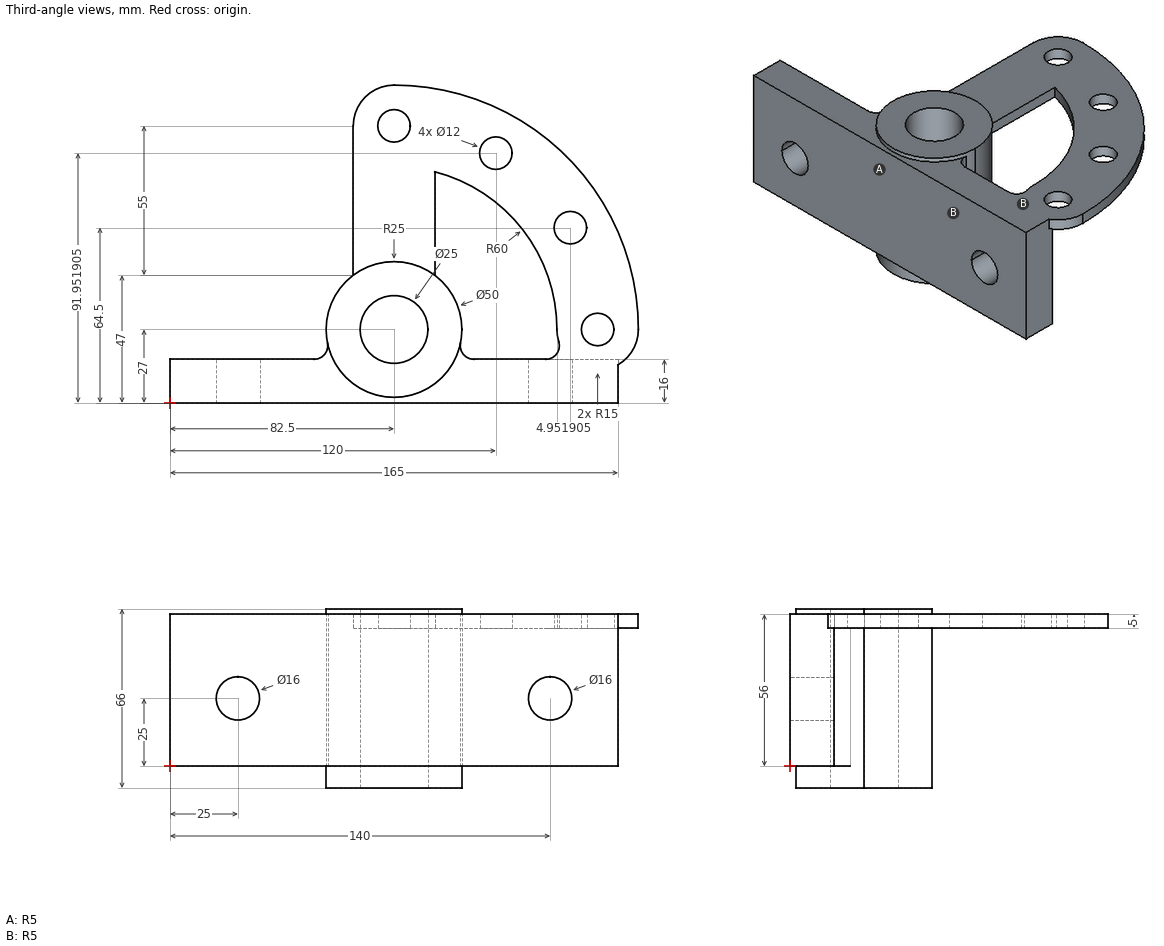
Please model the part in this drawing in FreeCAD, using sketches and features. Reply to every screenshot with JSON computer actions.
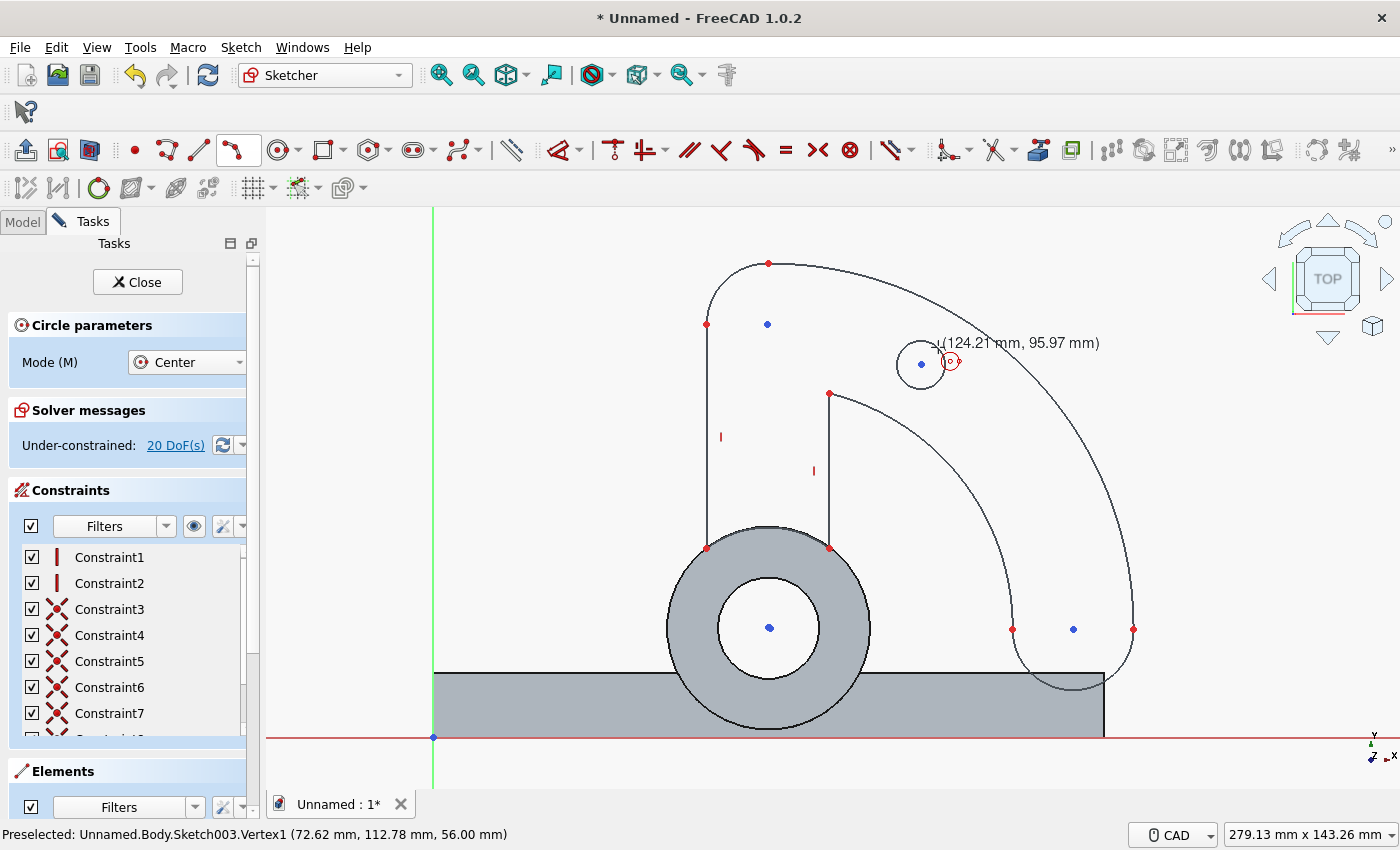
{"action": "left_click", "coordinate": [769, 324]}
{"action": "left_click", "coordinate": [786, 306]}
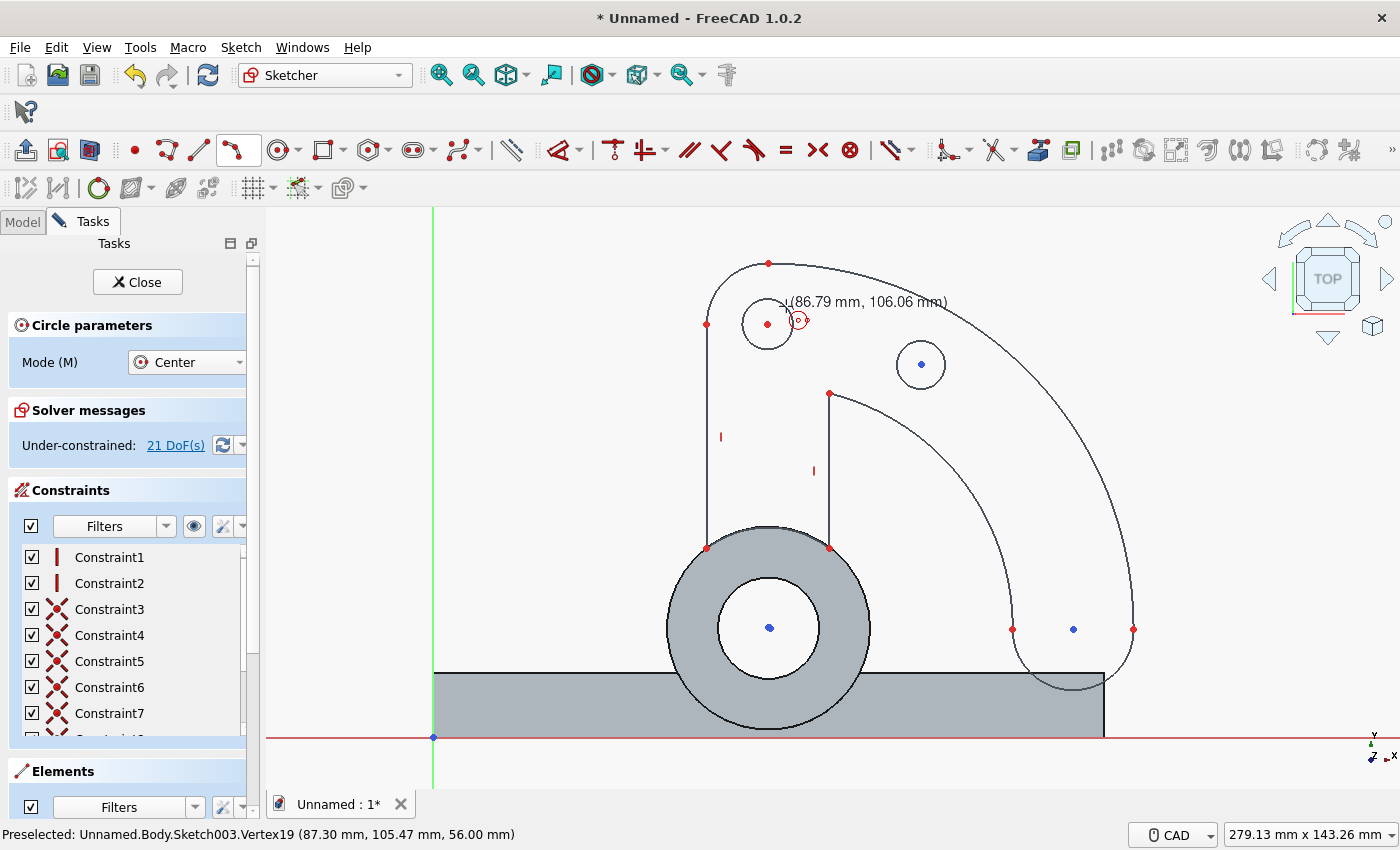
{"action": "left_click", "coordinate": [1073, 628]}
{"action": "left_click", "coordinate": [1090, 611]}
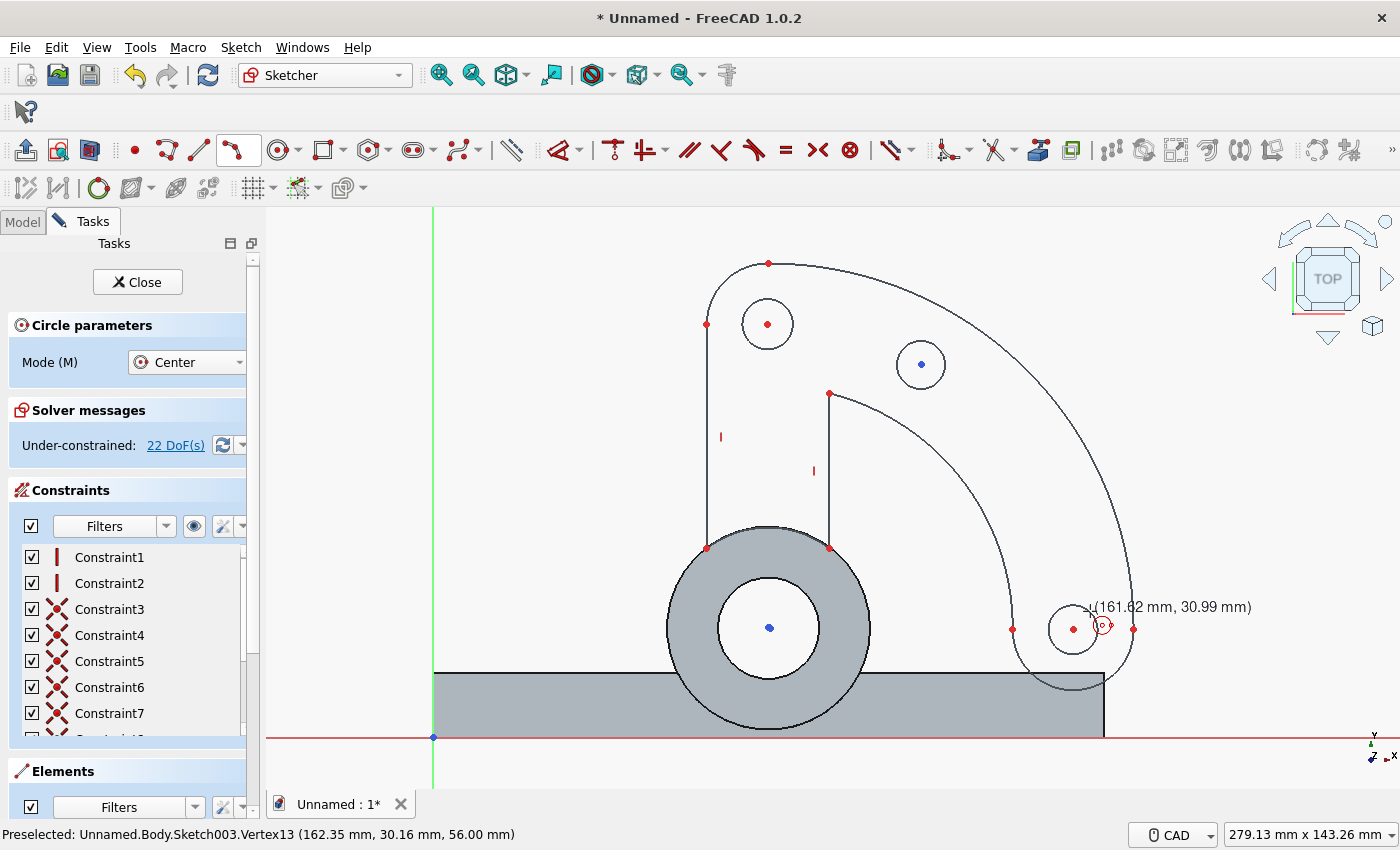
{"action": "left_click", "coordinate": [1032, 476]}
{"action": "left_click", "coordinate": [1050, 459]}
{"action": "key", "text": "Escape"}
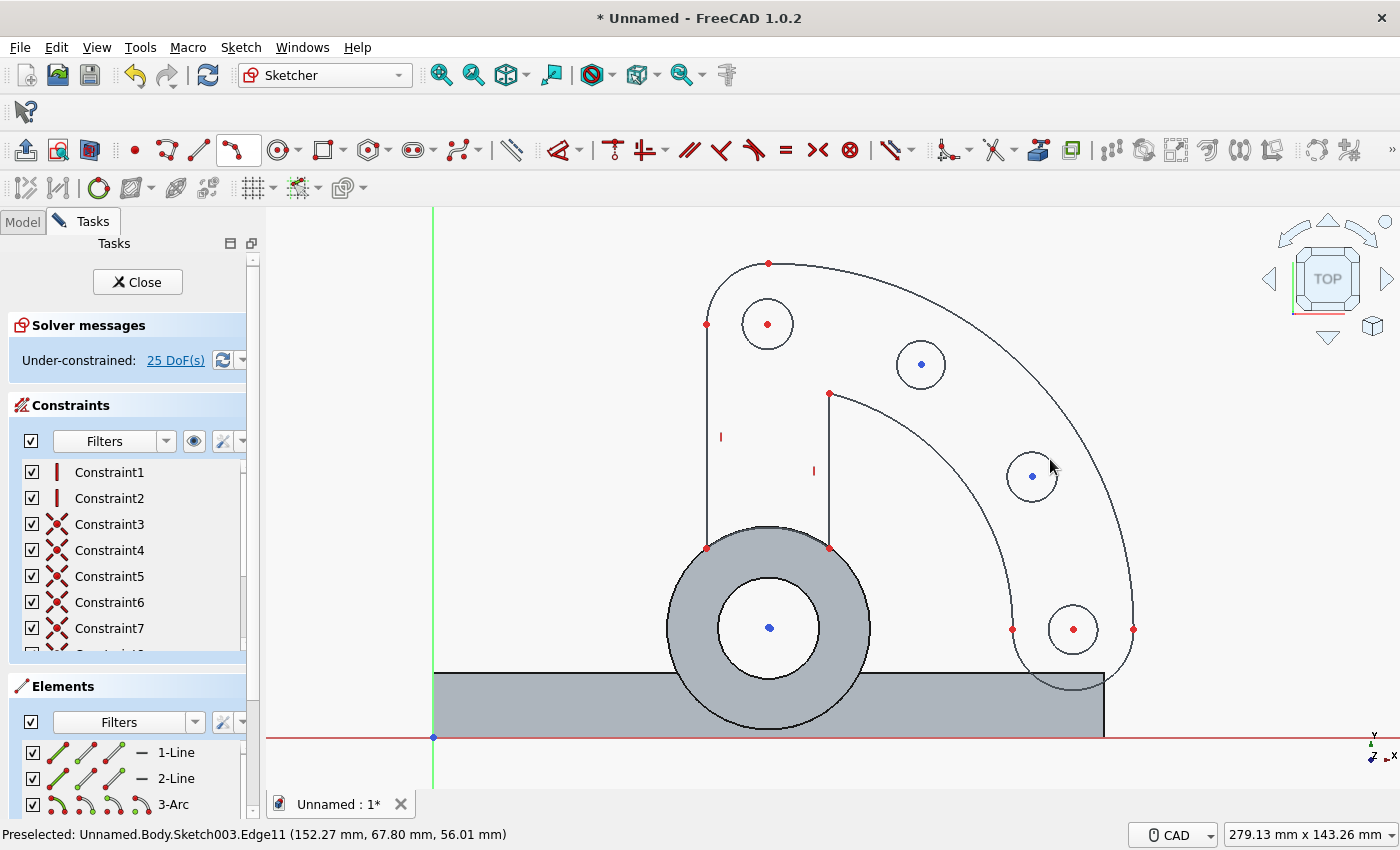
{"action": "left_click", "coordinate": [707, 392]}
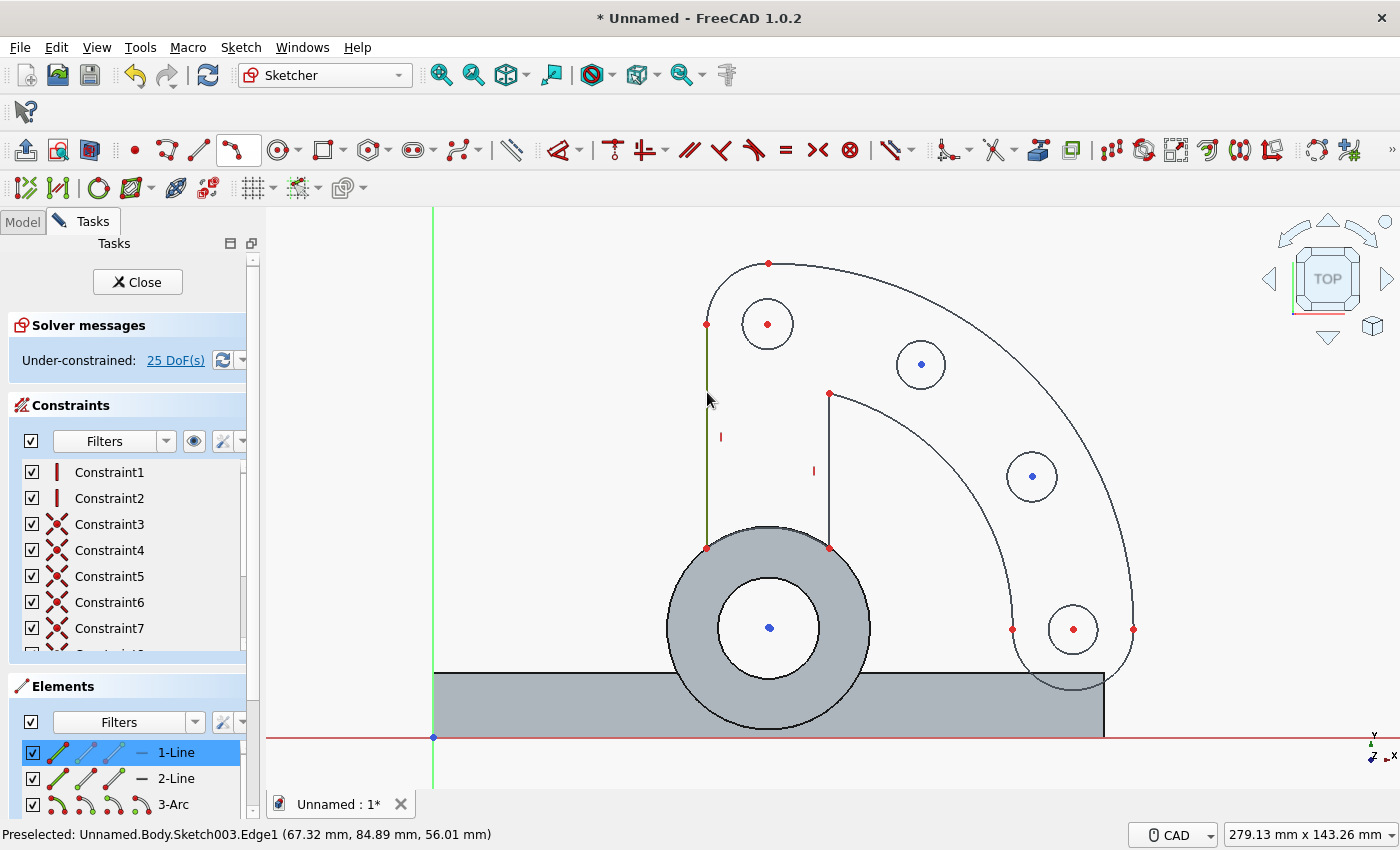
{"action": "left_click", "coordinate": [740, 270]}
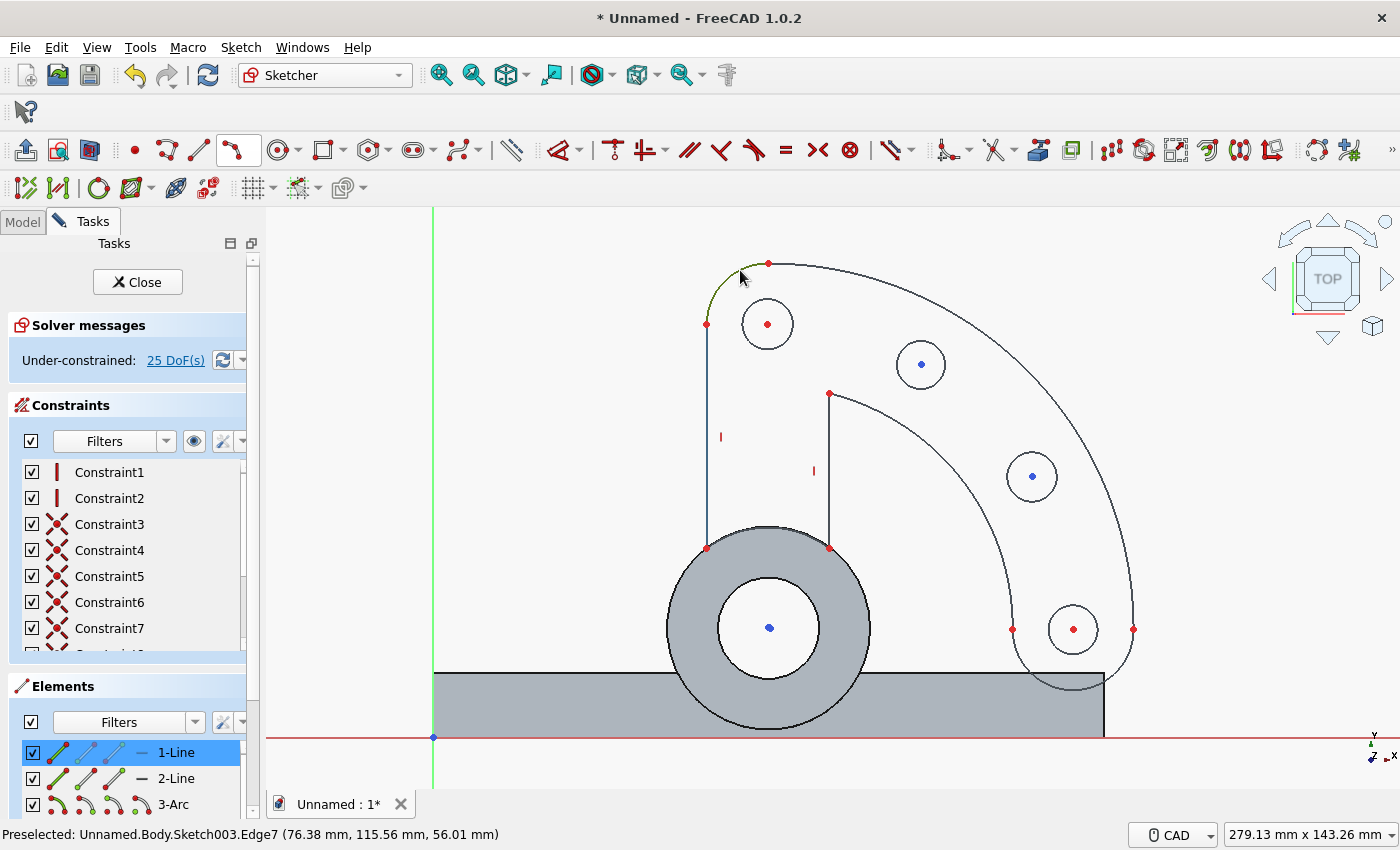
{"action": "left_click", "coordinate": [754, 150]}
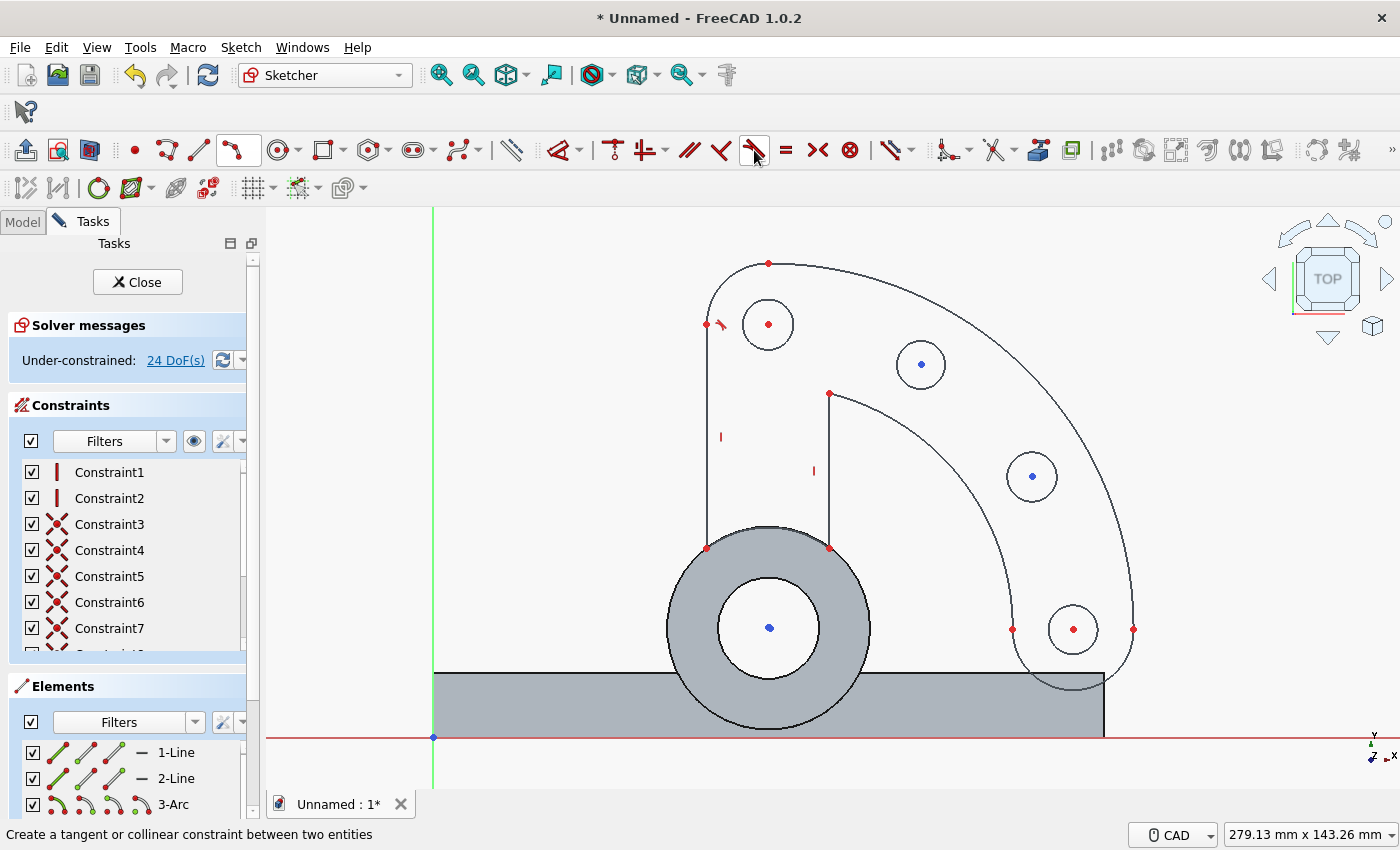
{"action": "left_click", "coordinate": [994, 535]}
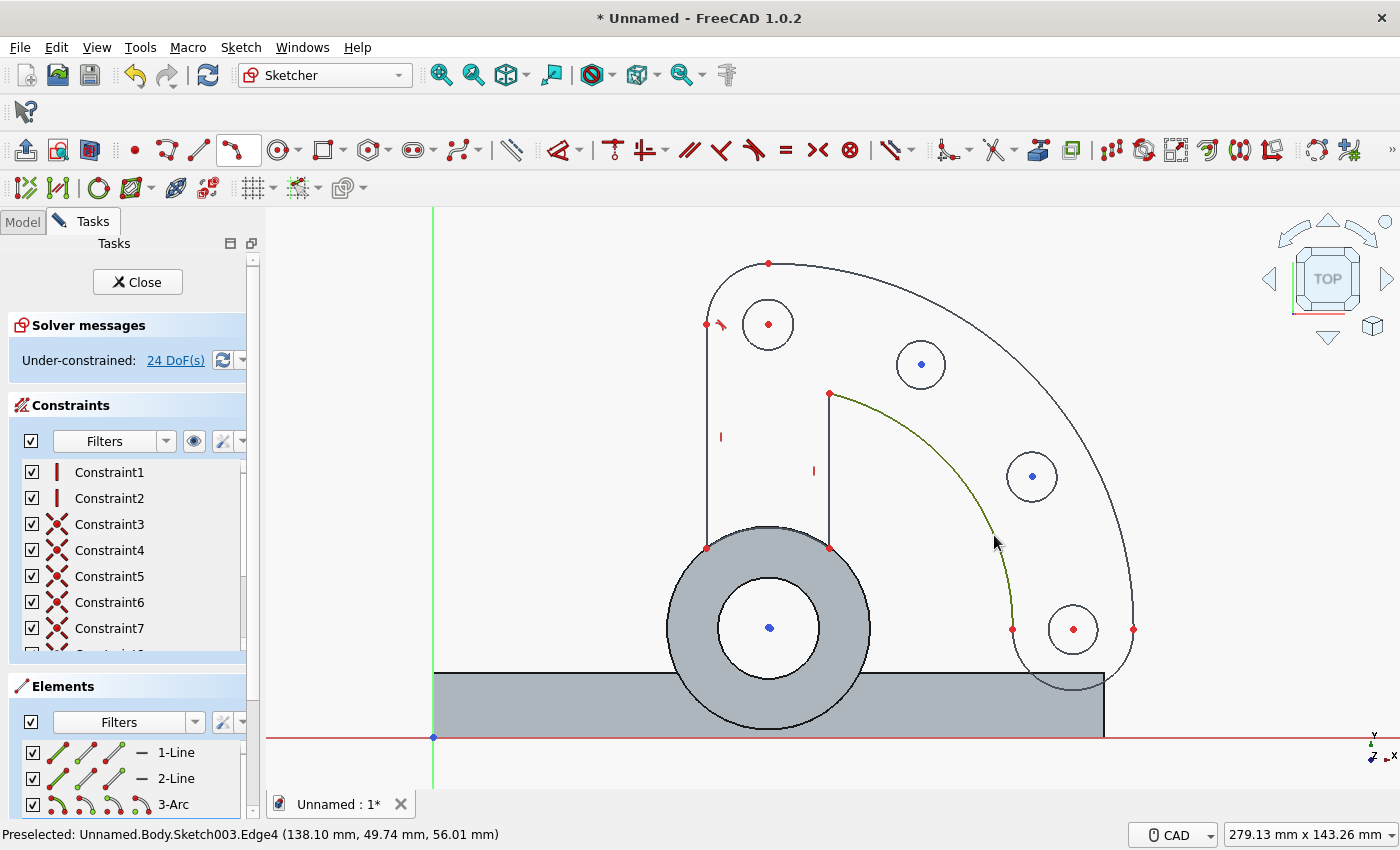
{"action": "left_click", "coordinate": [1037, 678]}